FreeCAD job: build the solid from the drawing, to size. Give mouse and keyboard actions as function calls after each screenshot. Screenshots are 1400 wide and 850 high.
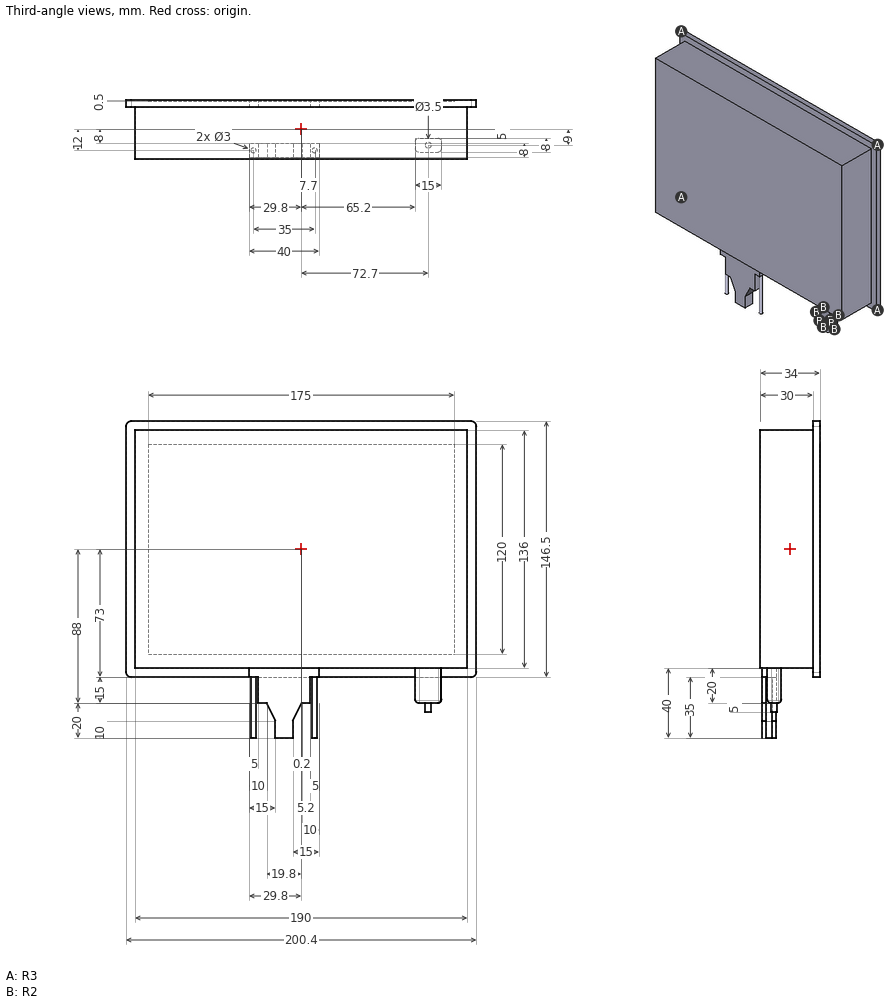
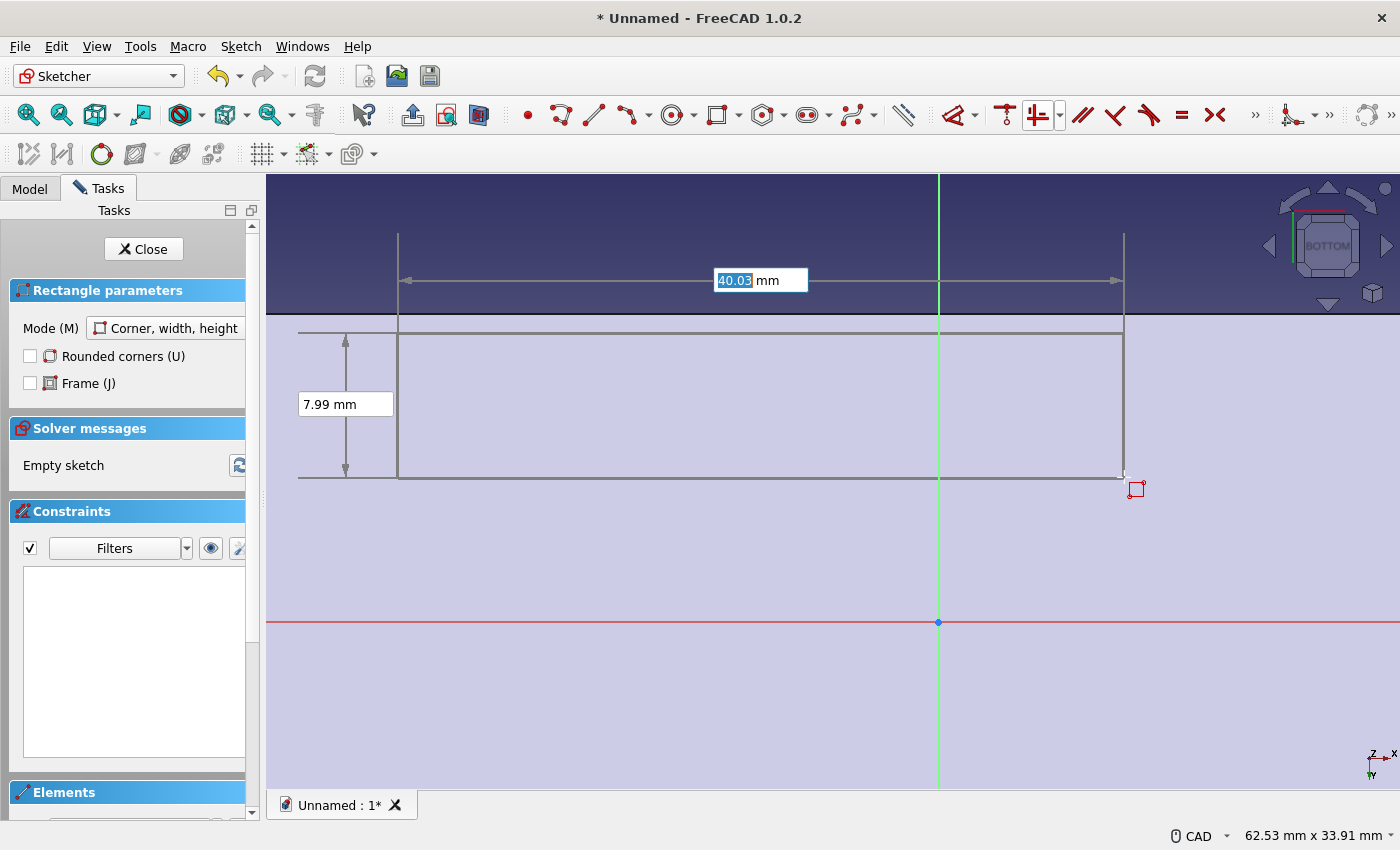
text(40)
key(Tab)
text(8)
key(Return)
key(Escape)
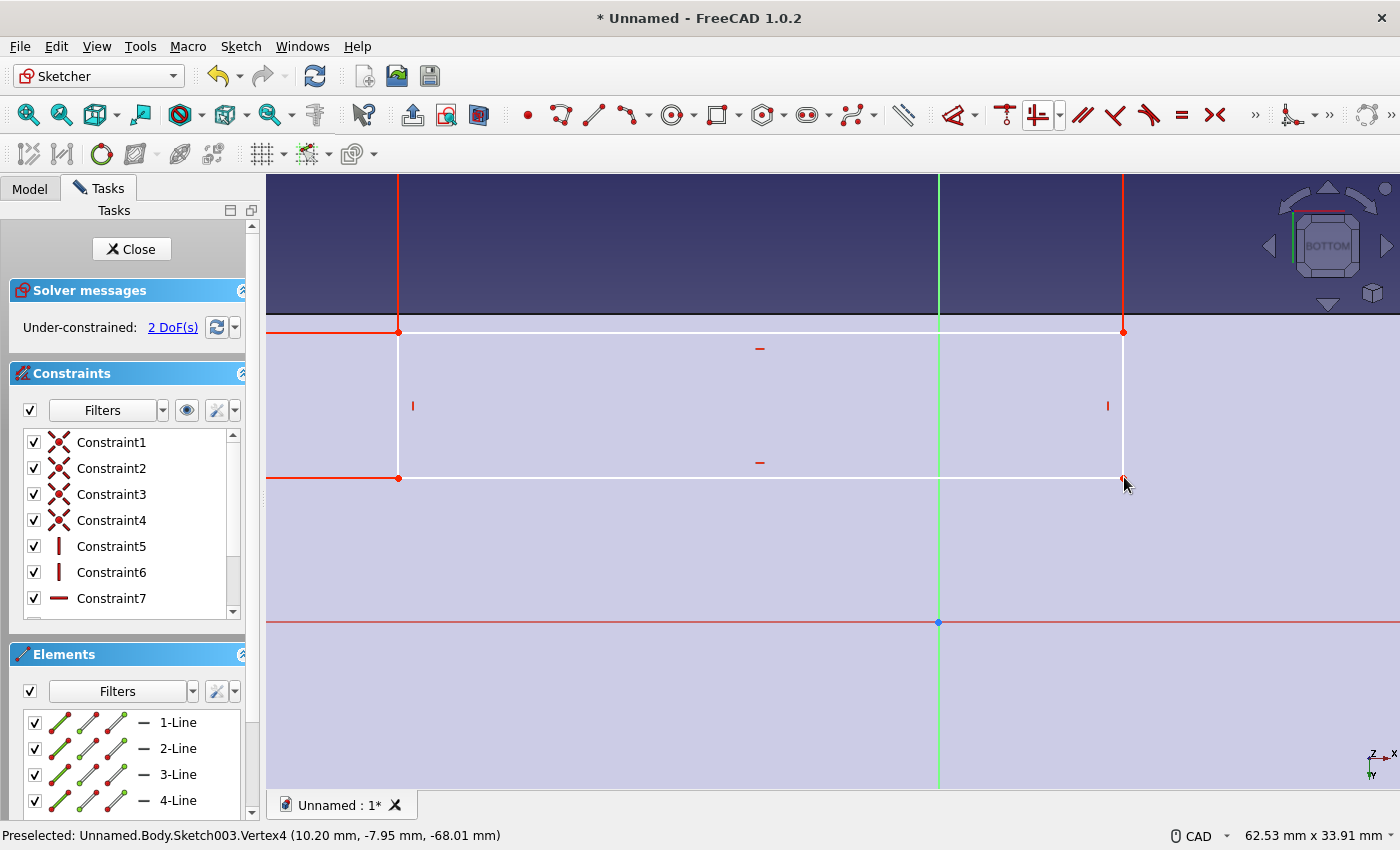
click(952, 116)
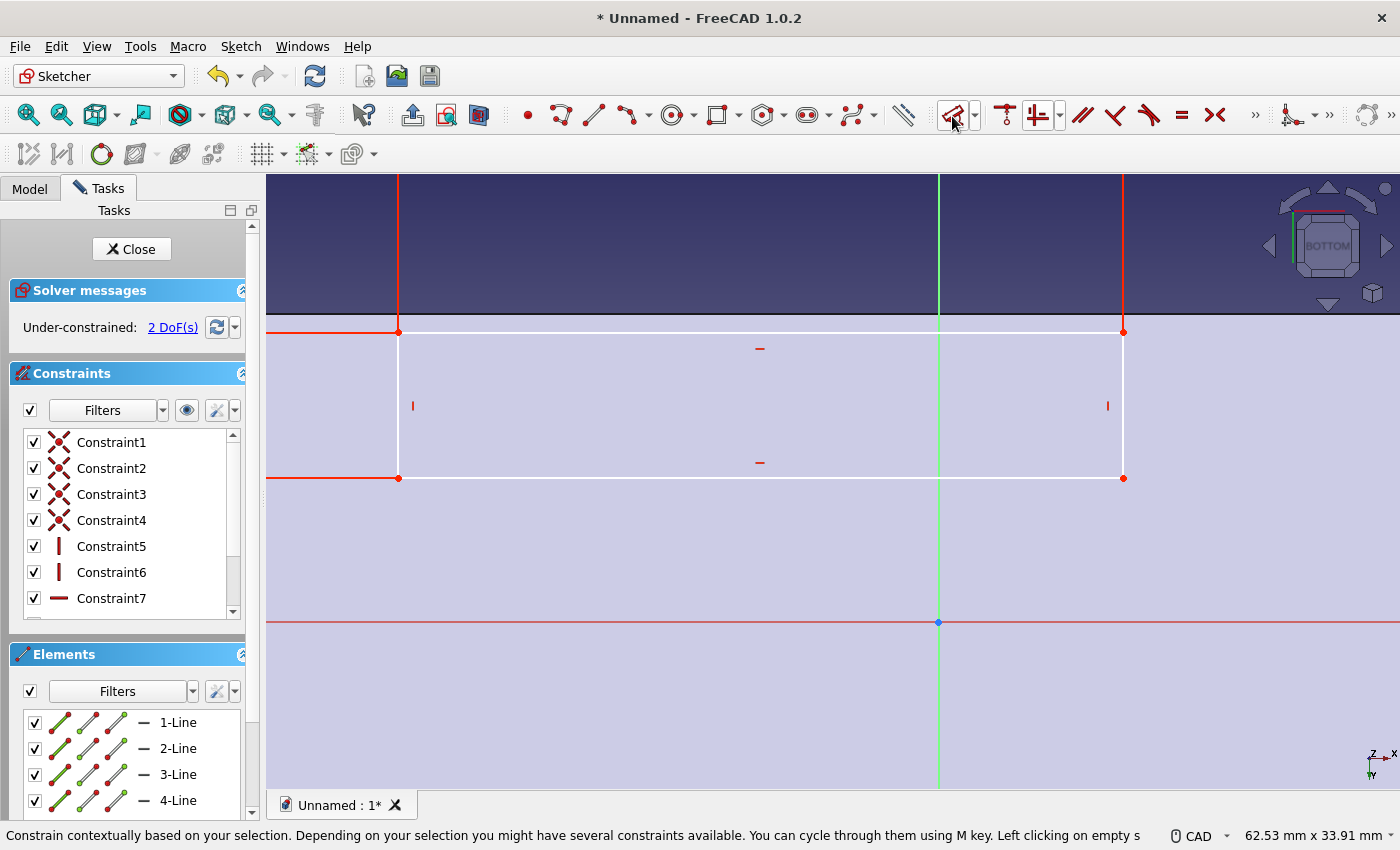
click(398, 478)
click(364, 550)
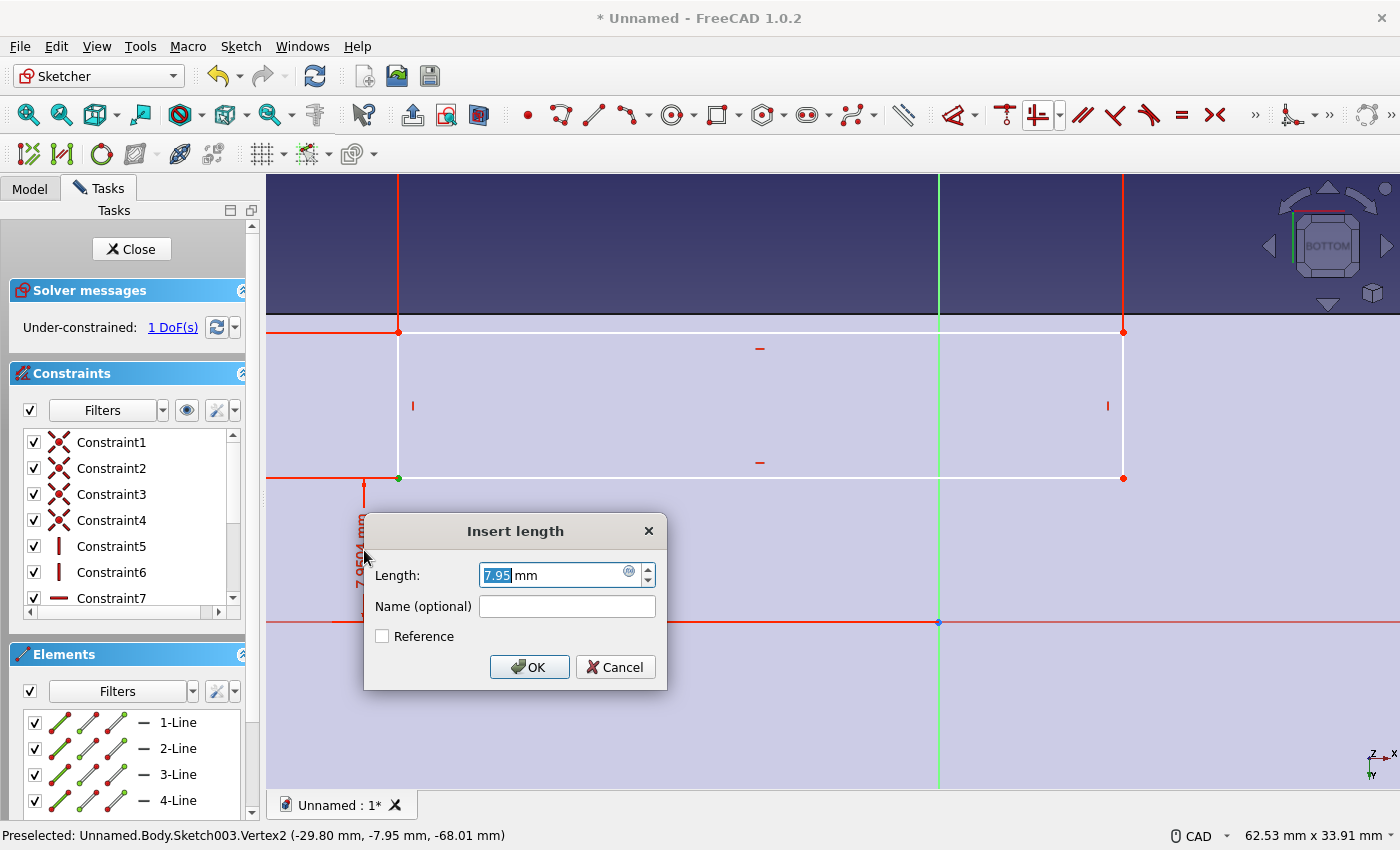
text(8)
key(Return)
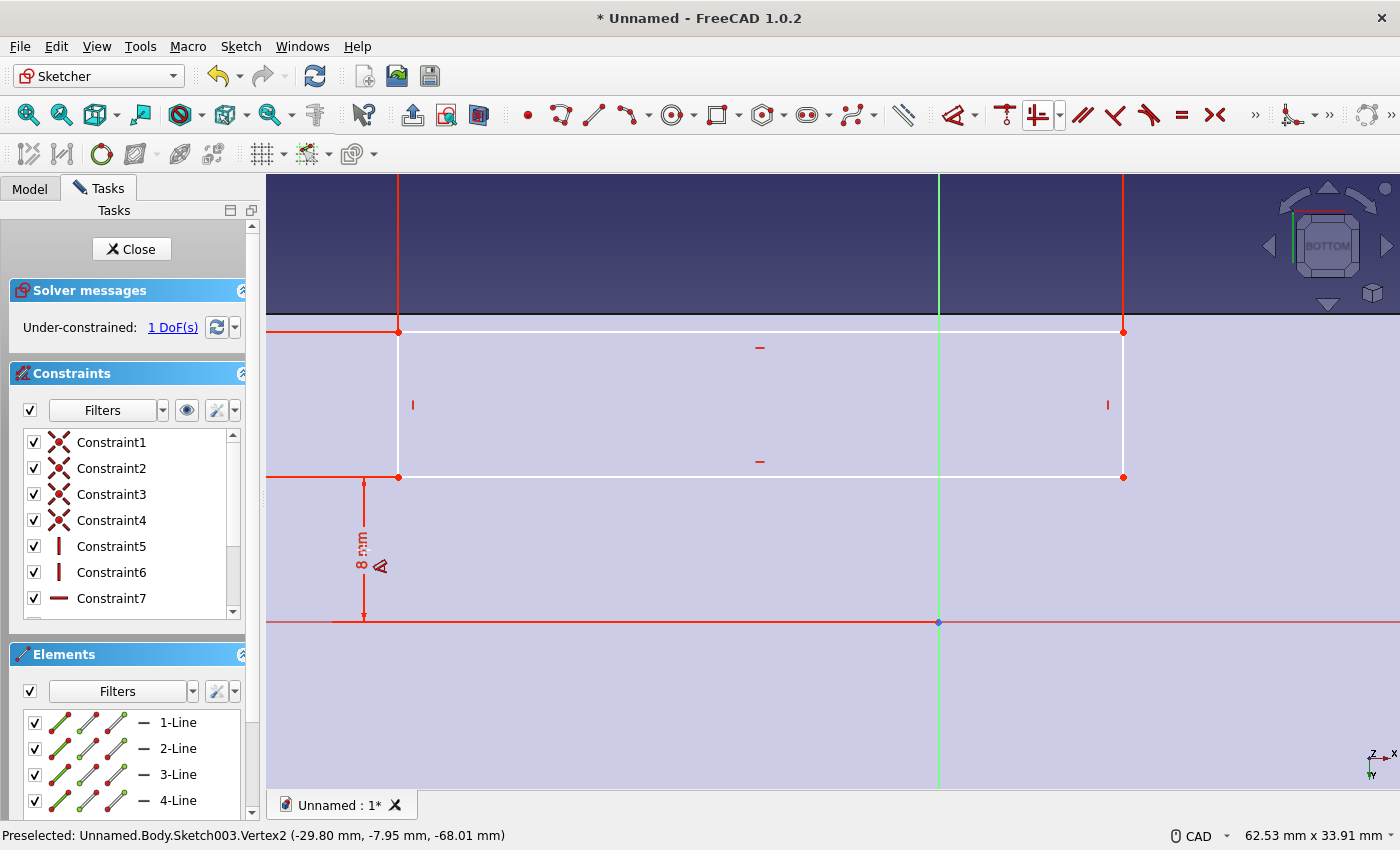
click(398, 332)
click(668, 656)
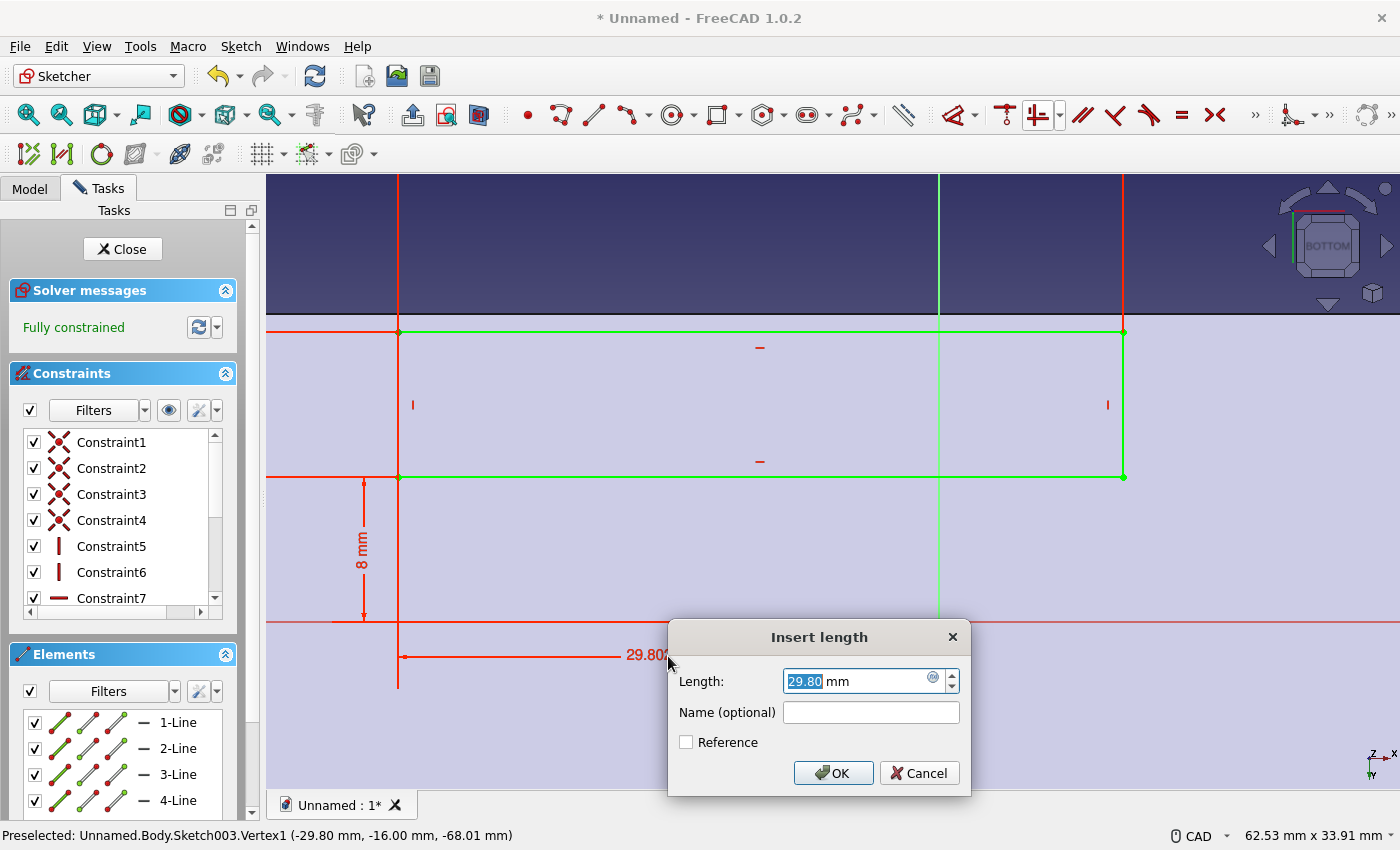
text(29.8)
key(Return)
key(Escape)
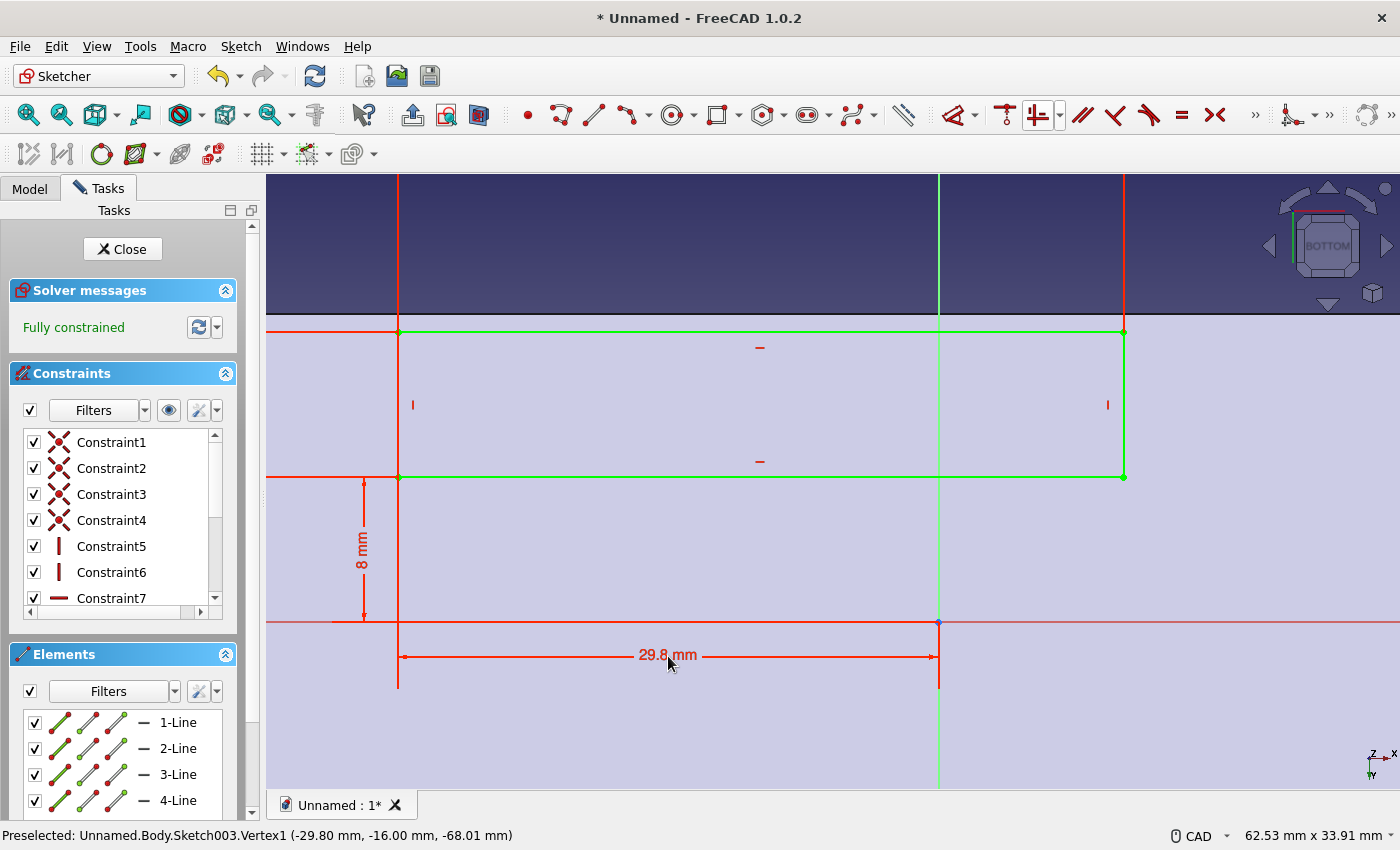
click(123, 249)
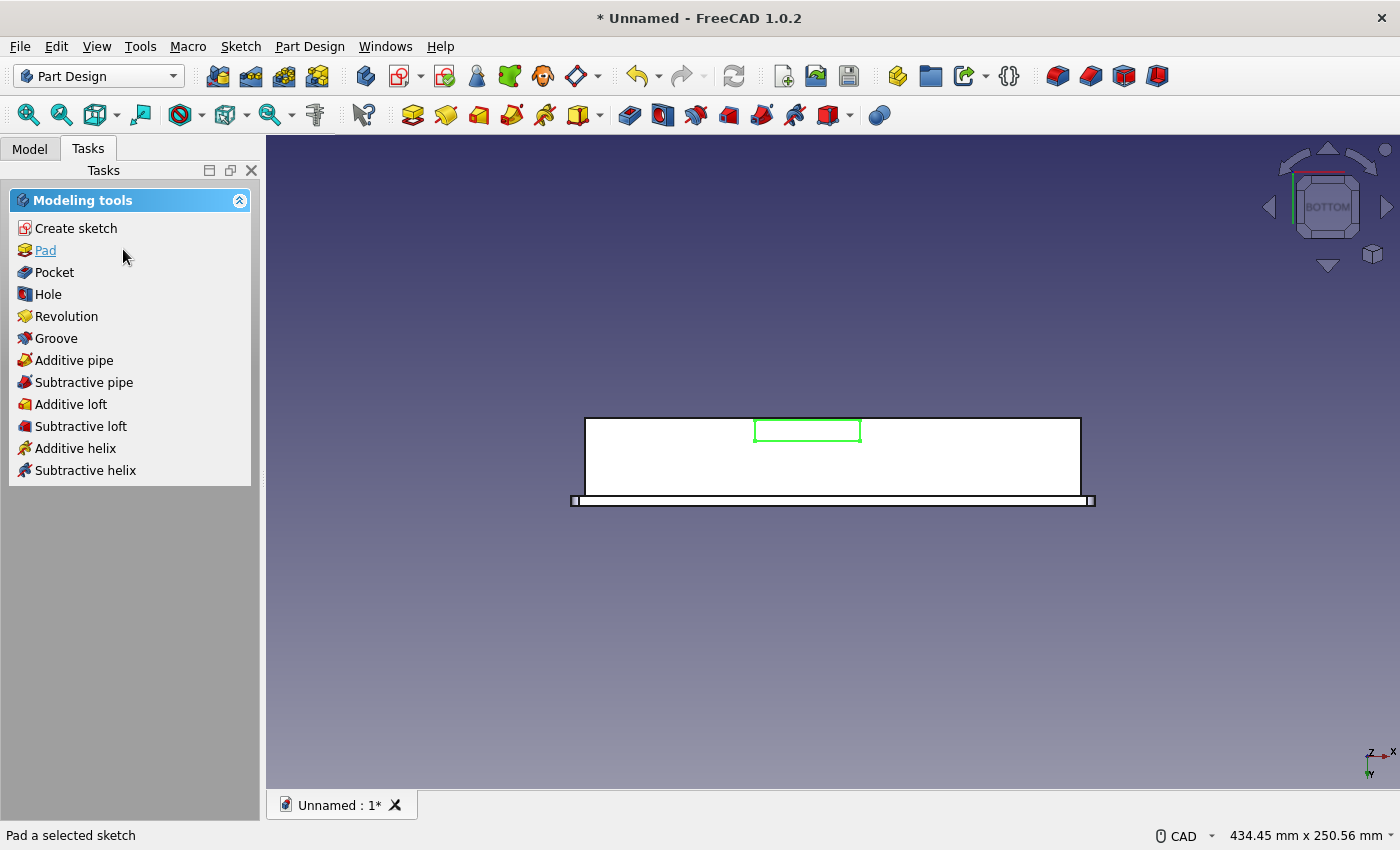
click(413, 116)